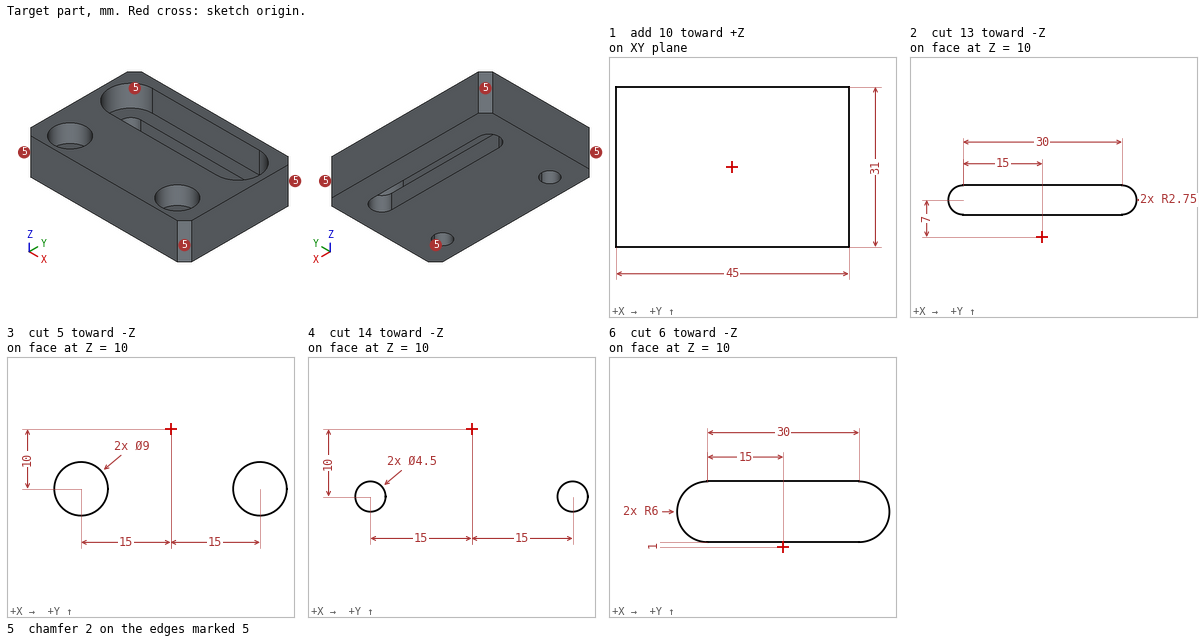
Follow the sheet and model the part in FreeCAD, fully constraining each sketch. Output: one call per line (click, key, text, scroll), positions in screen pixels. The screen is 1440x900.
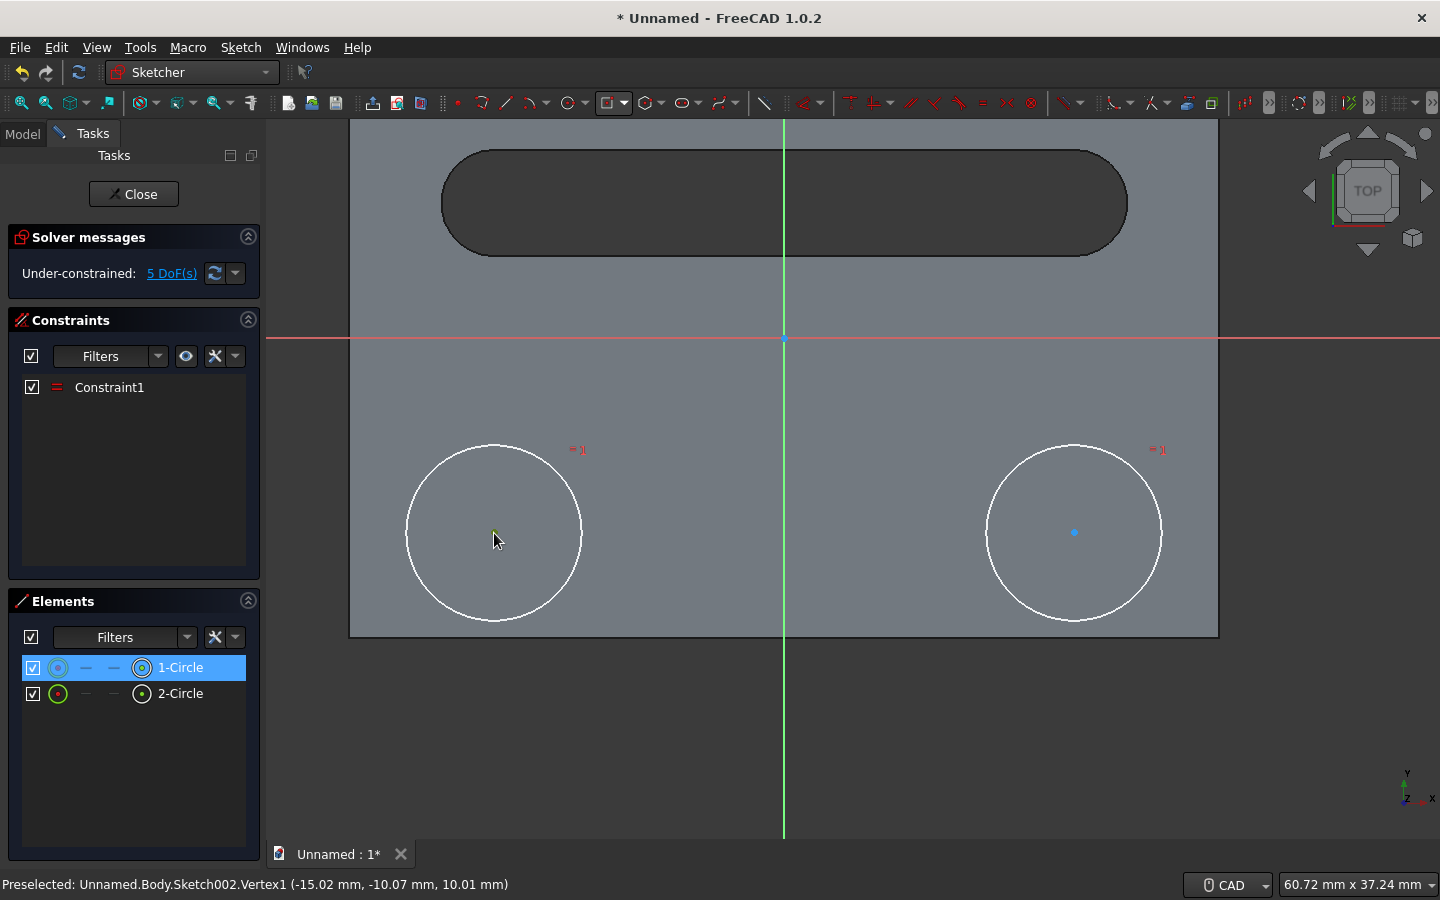
click(1074, 533)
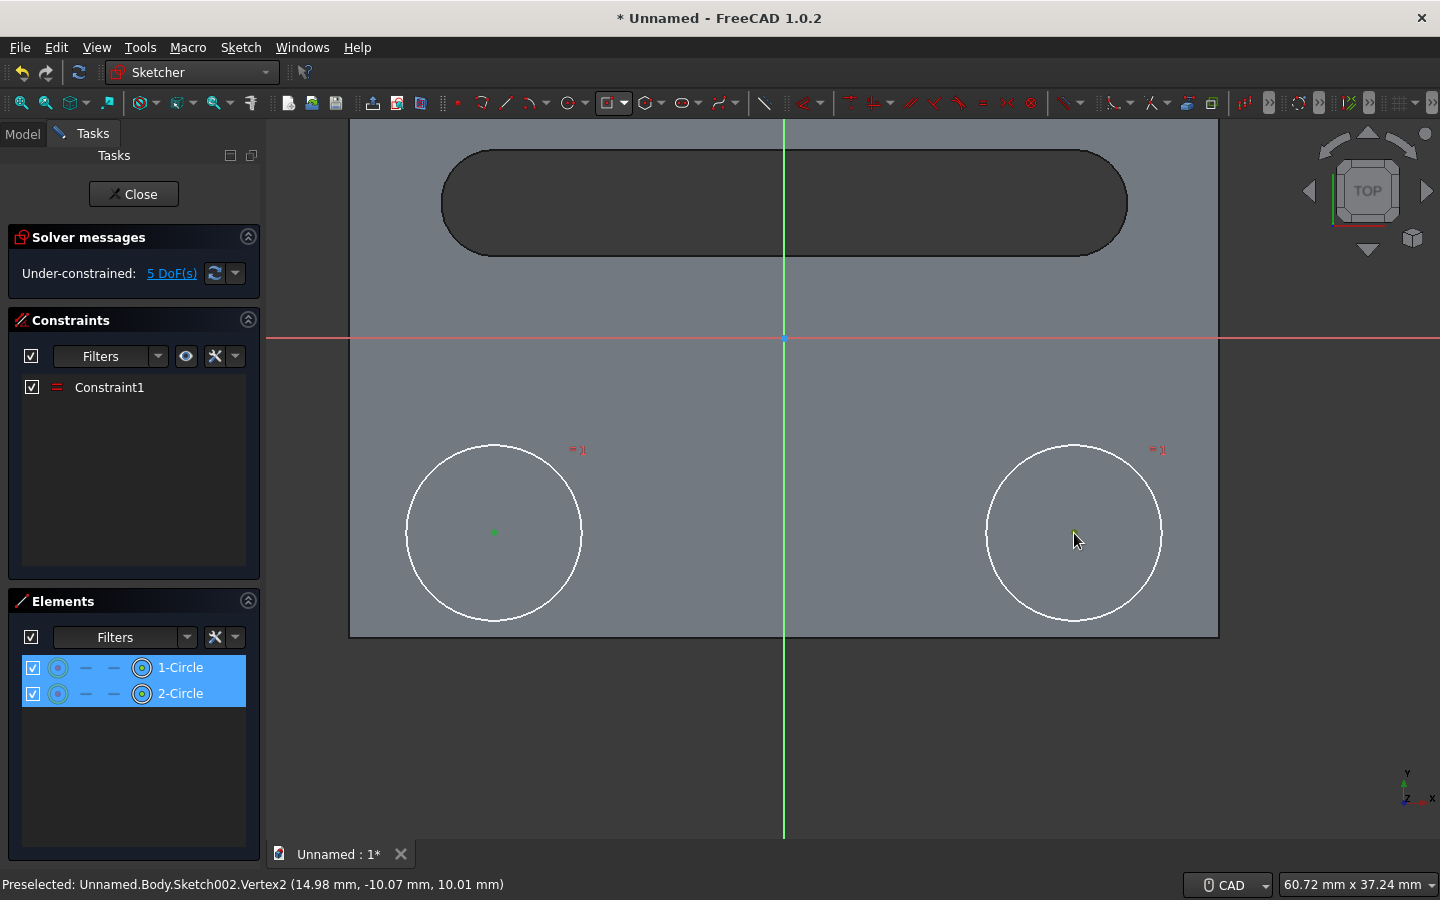
key(h)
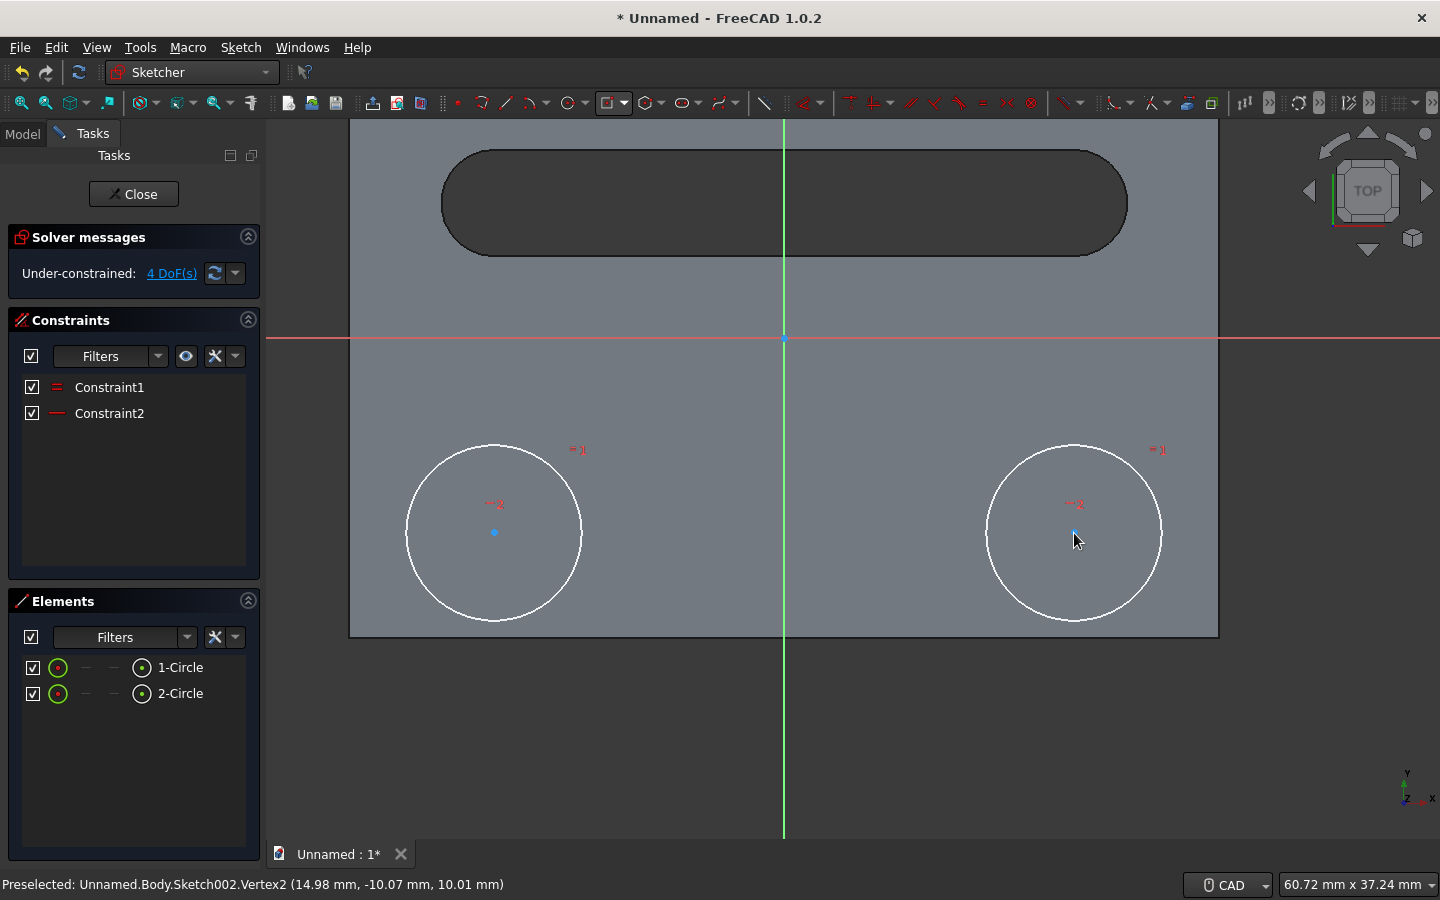
click(804, 104)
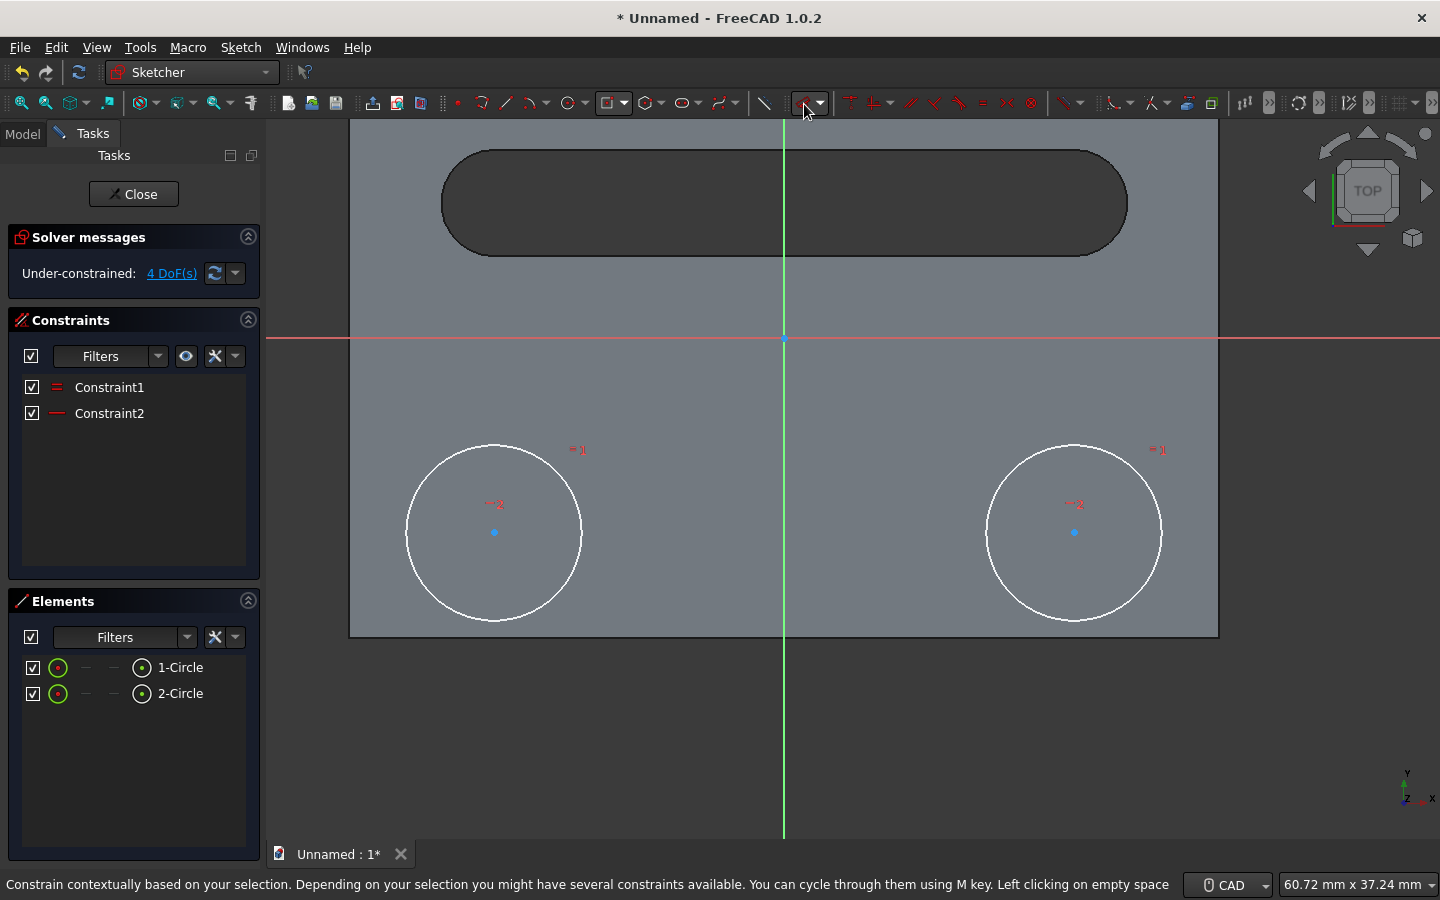
click(556, 471)
click(579, 448)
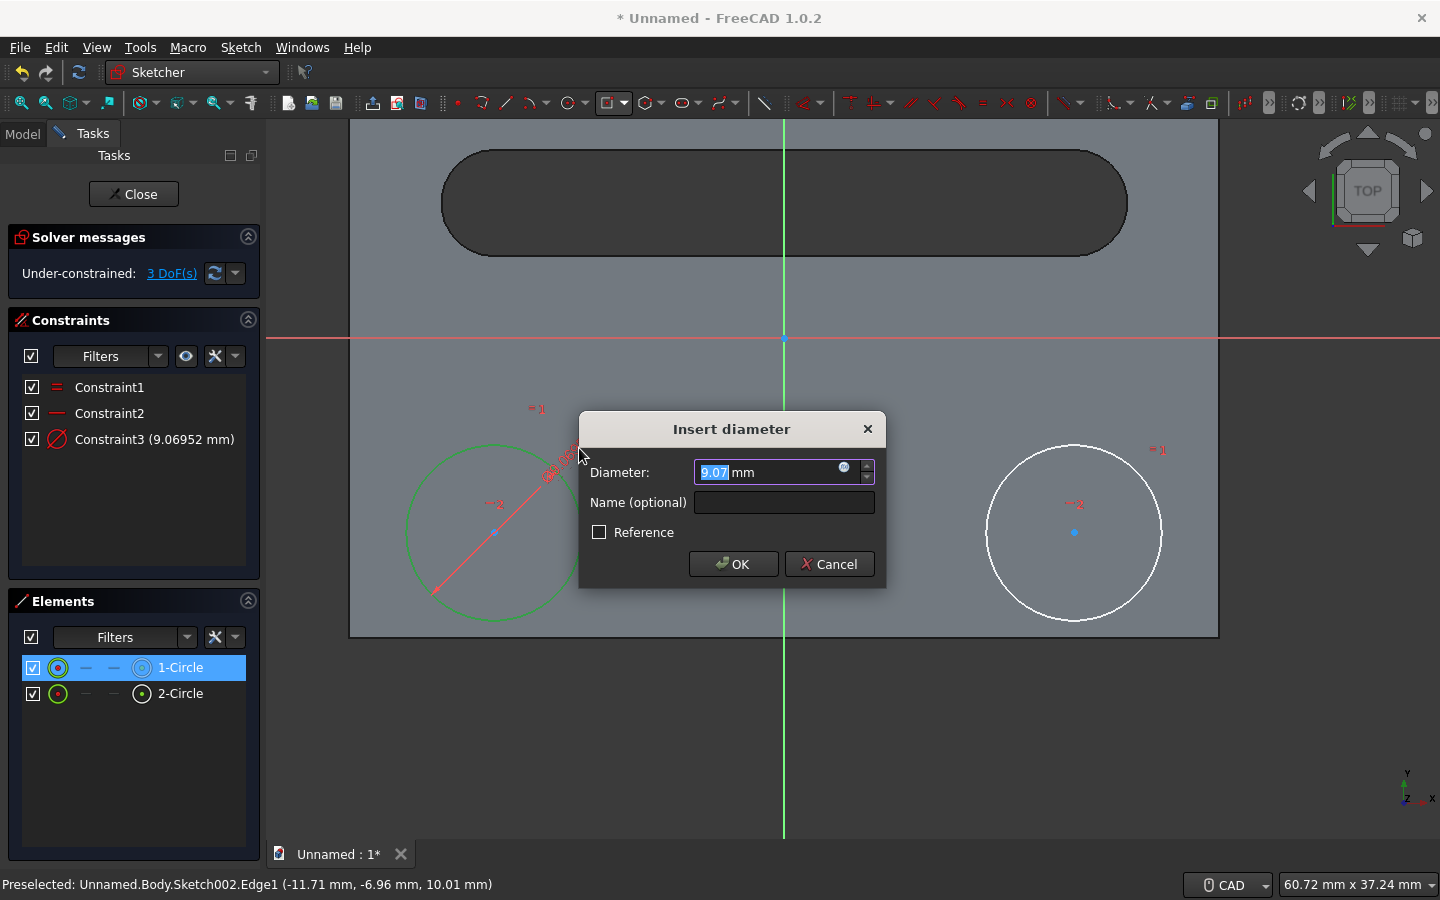
text(9)
key(Return)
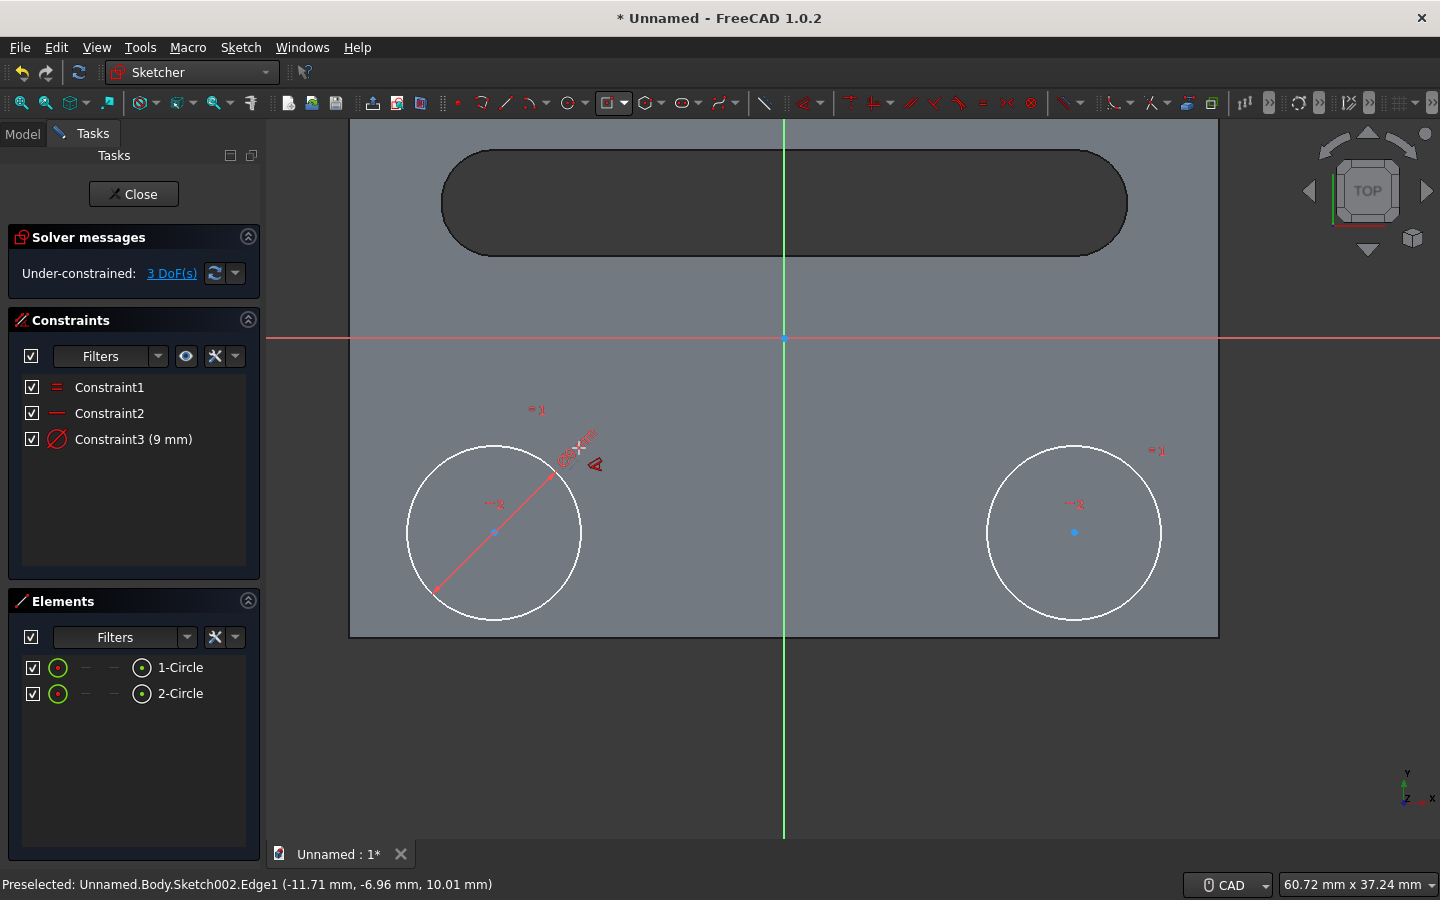
click(494, 533)
click(639, 304)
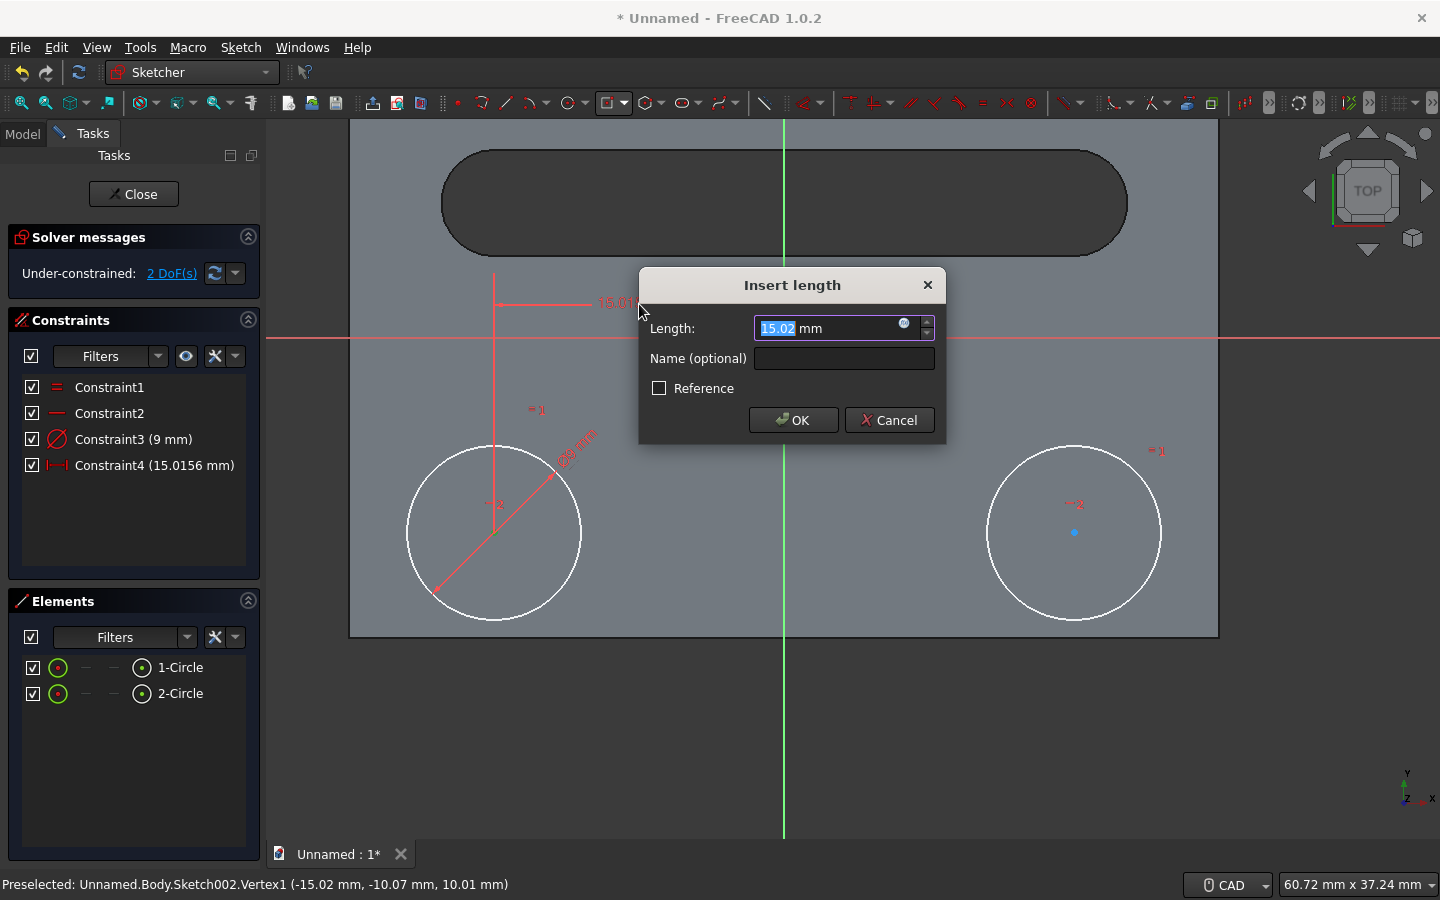
text(15)
key(Return)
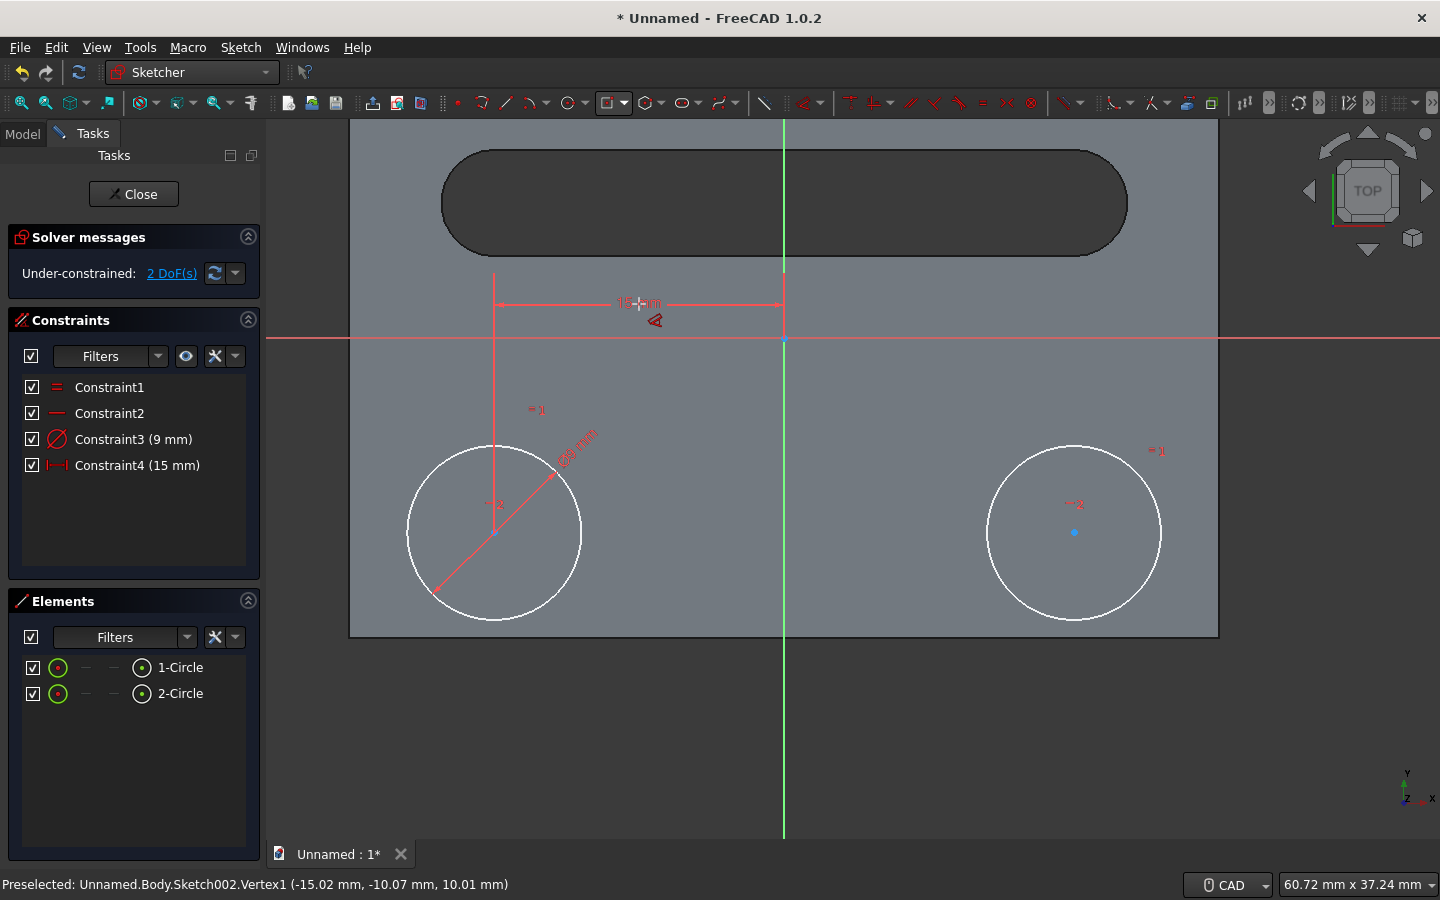
click(494, 533)
click(460, 436)